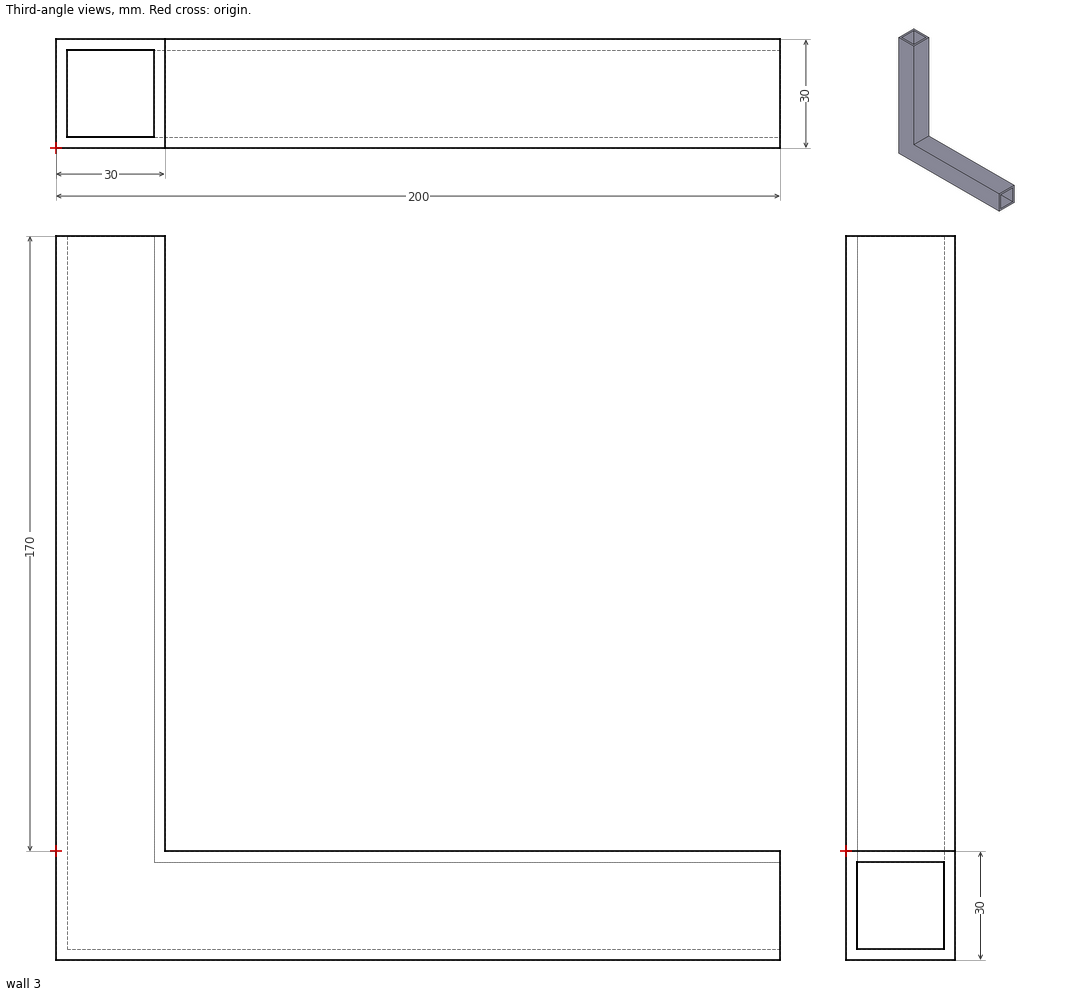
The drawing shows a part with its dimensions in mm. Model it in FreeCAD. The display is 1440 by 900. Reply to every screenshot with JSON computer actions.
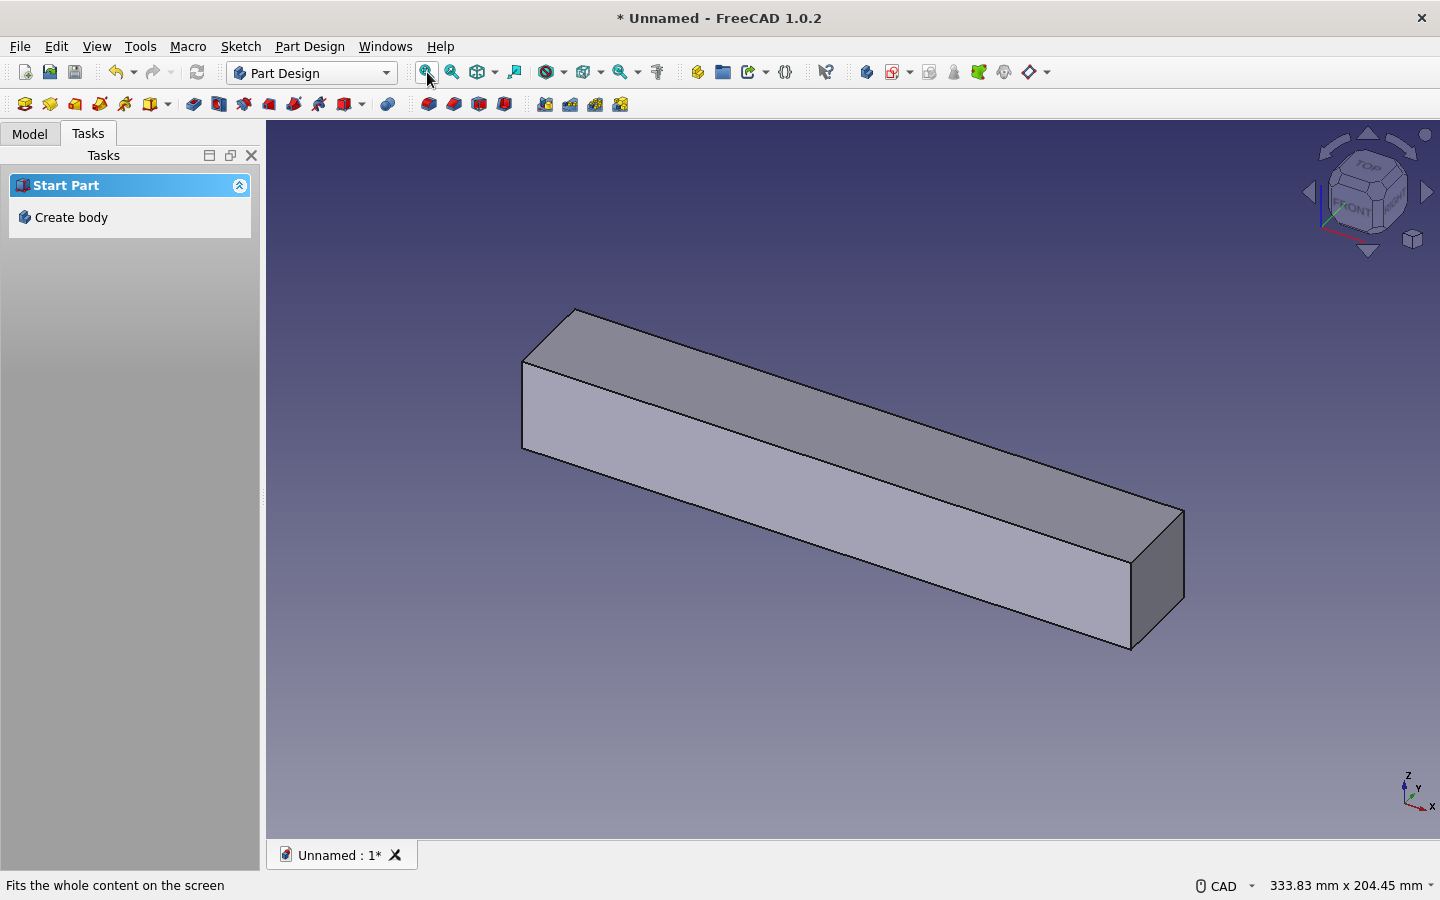
{"action": "left_click", "coordinate": [892, 72]}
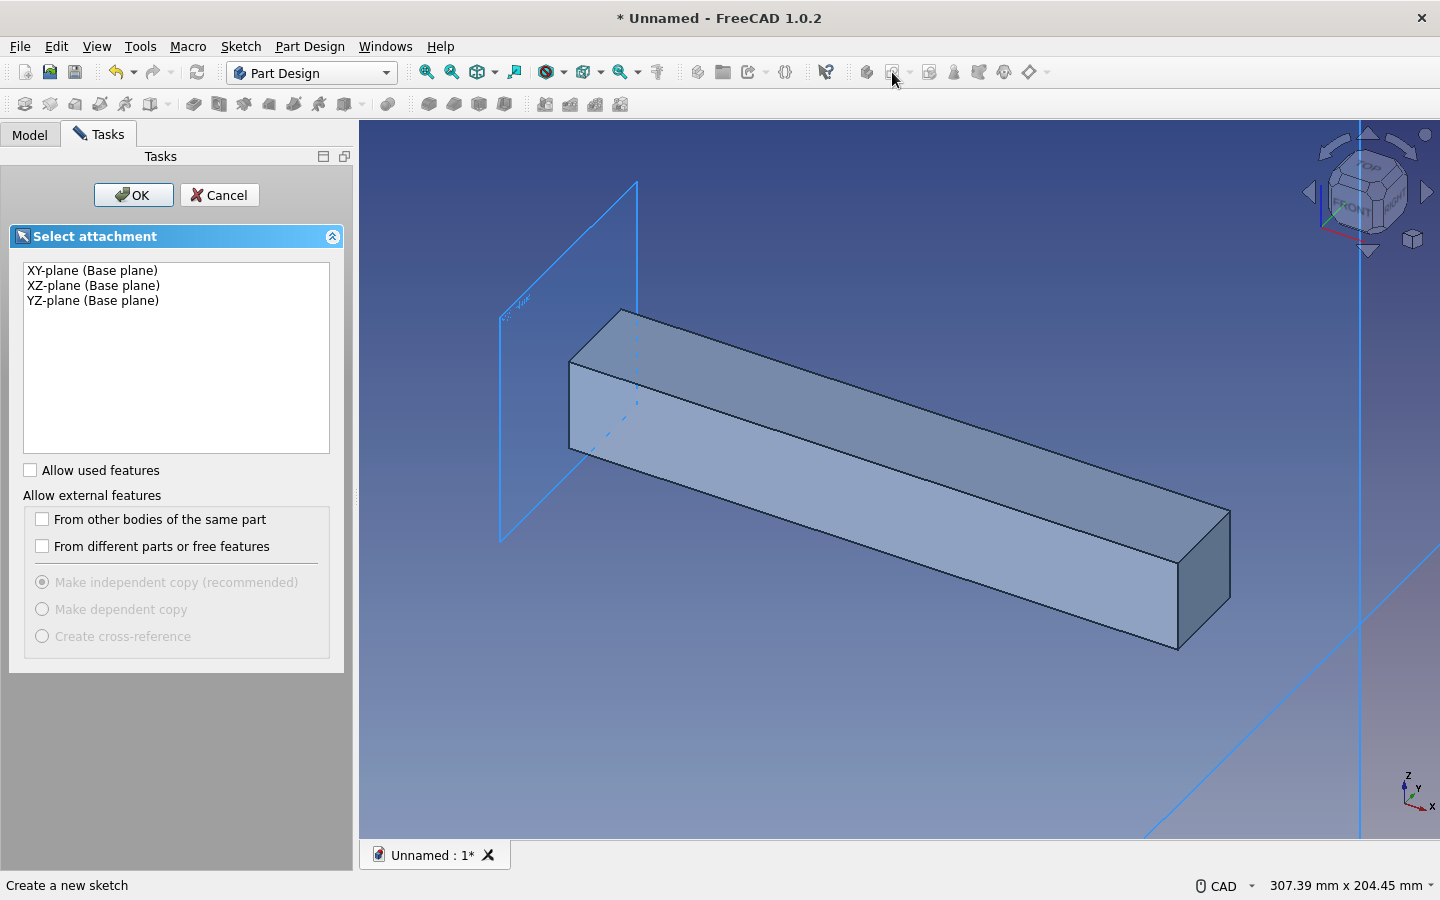
{"action": "left_click", "coordinate": [84, 270]}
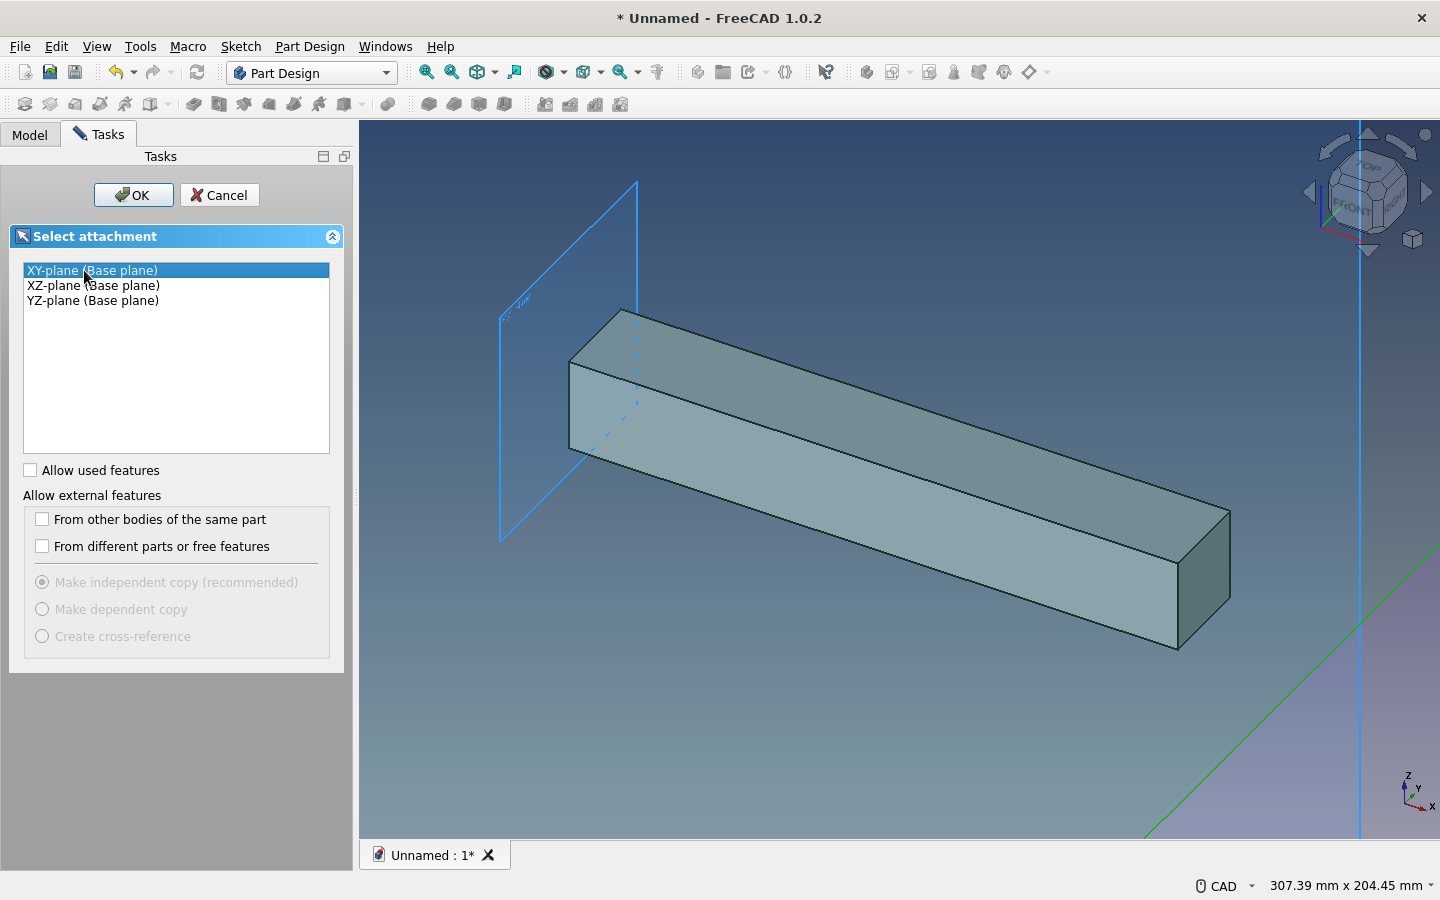
{"action": "left_click", "coordinate": [134, 195]}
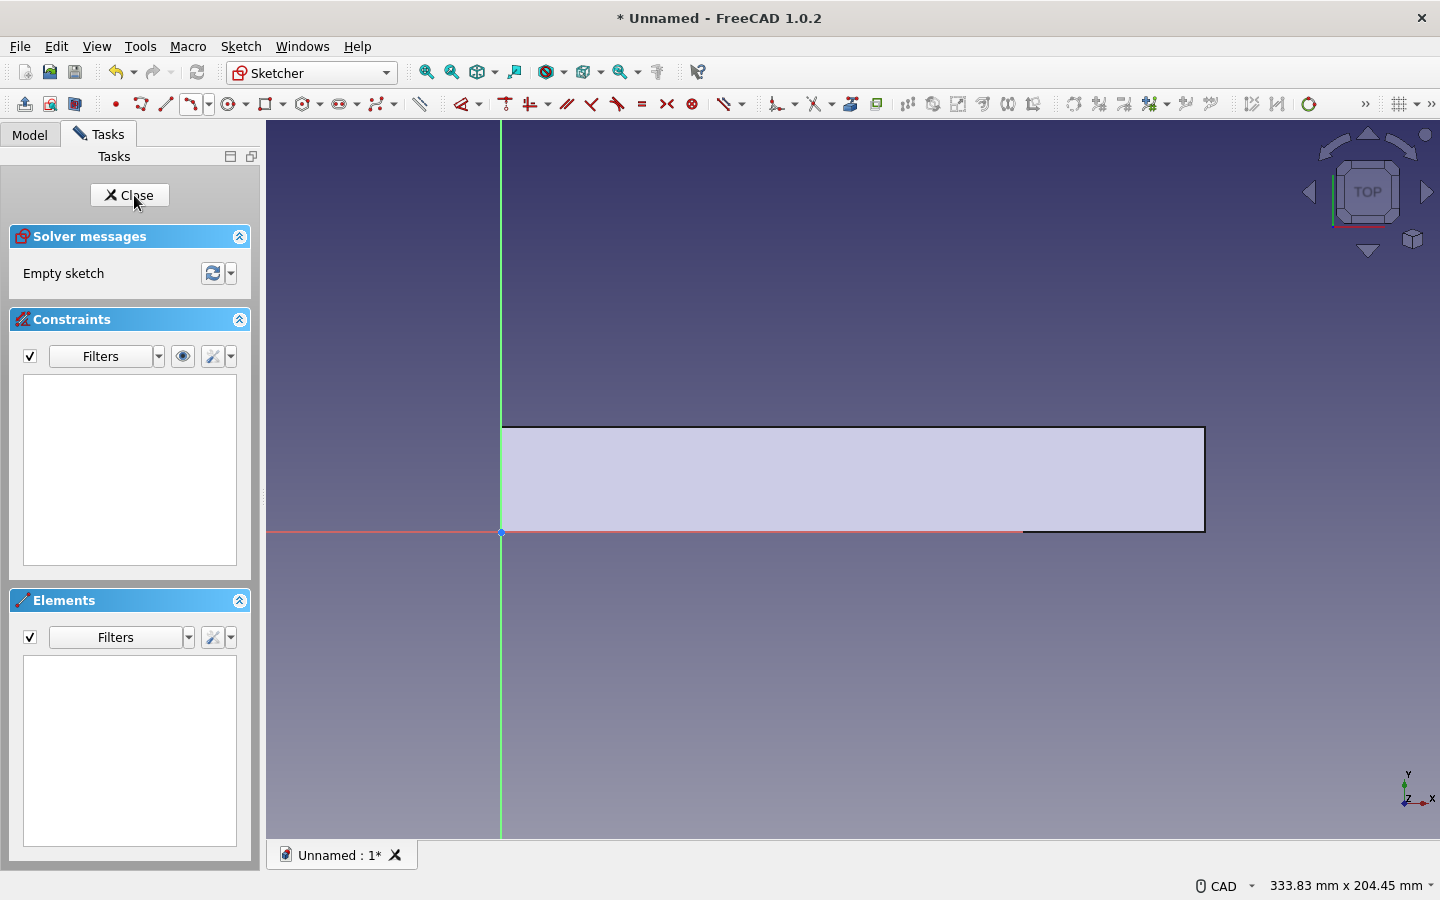
{"action": "scroll", "coordinate": [479, 480], "scroll_direction": "up", "scroll_amount": 7}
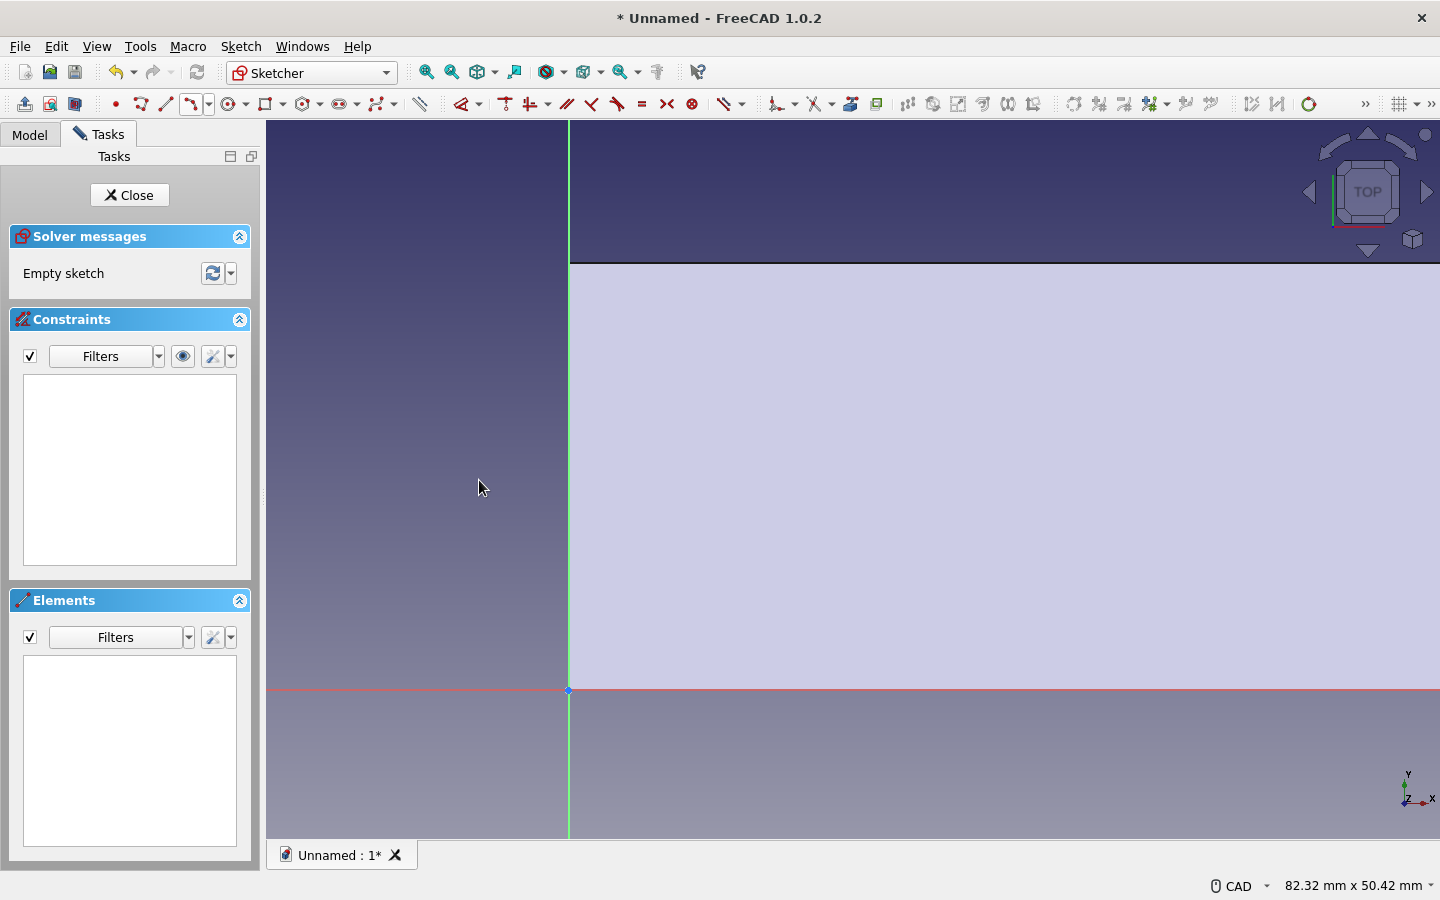
{"action": "left_click", "coordinate": [264, 104]}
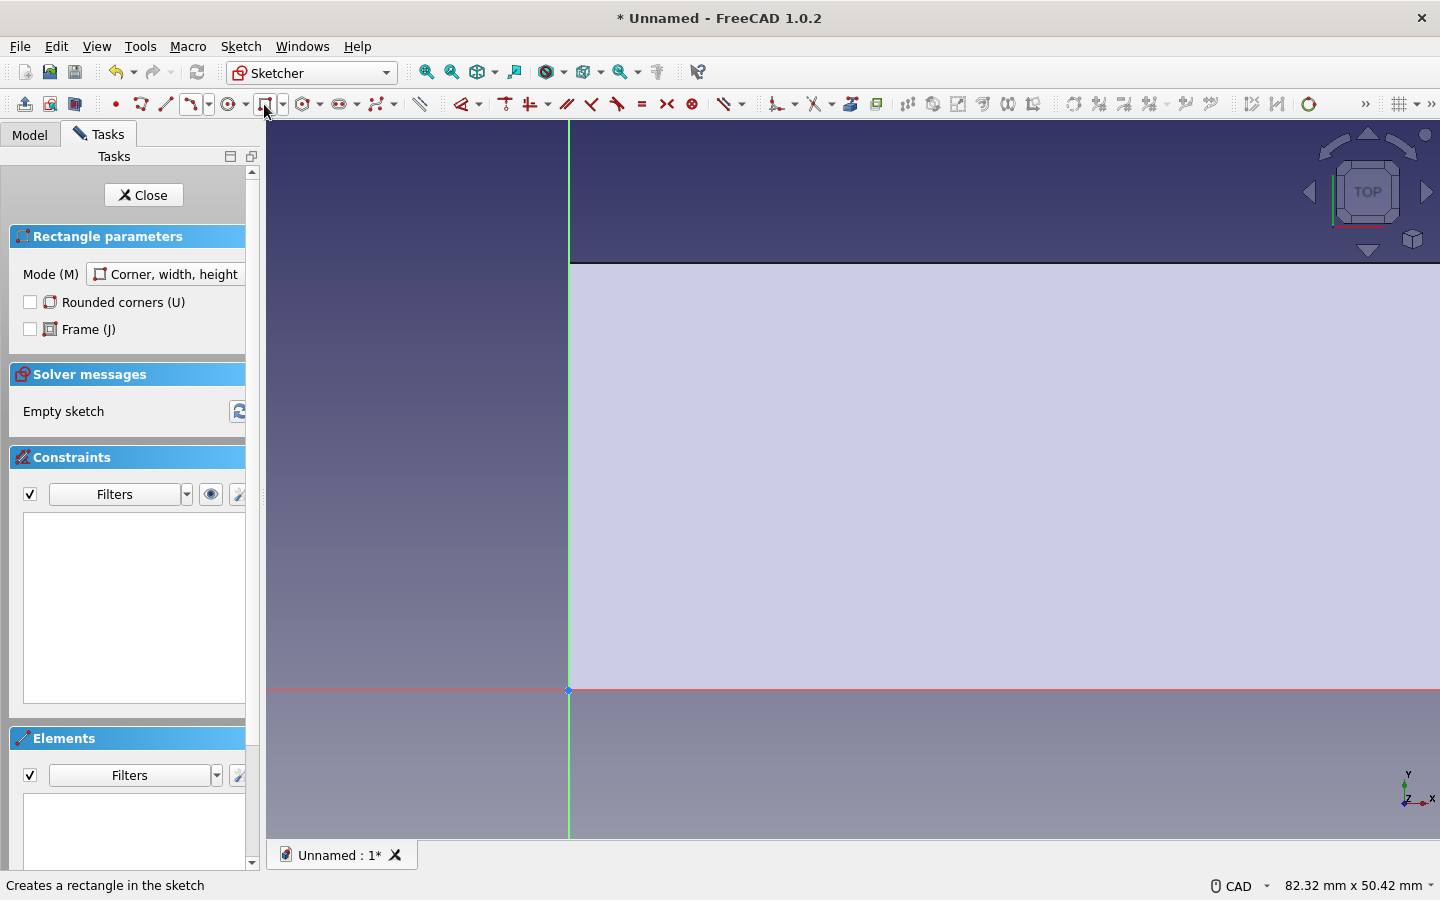
{"action": "left_click", "coordinate": [569, 690]}
{"action": "mouse_move", "coordinate": [997, 263]}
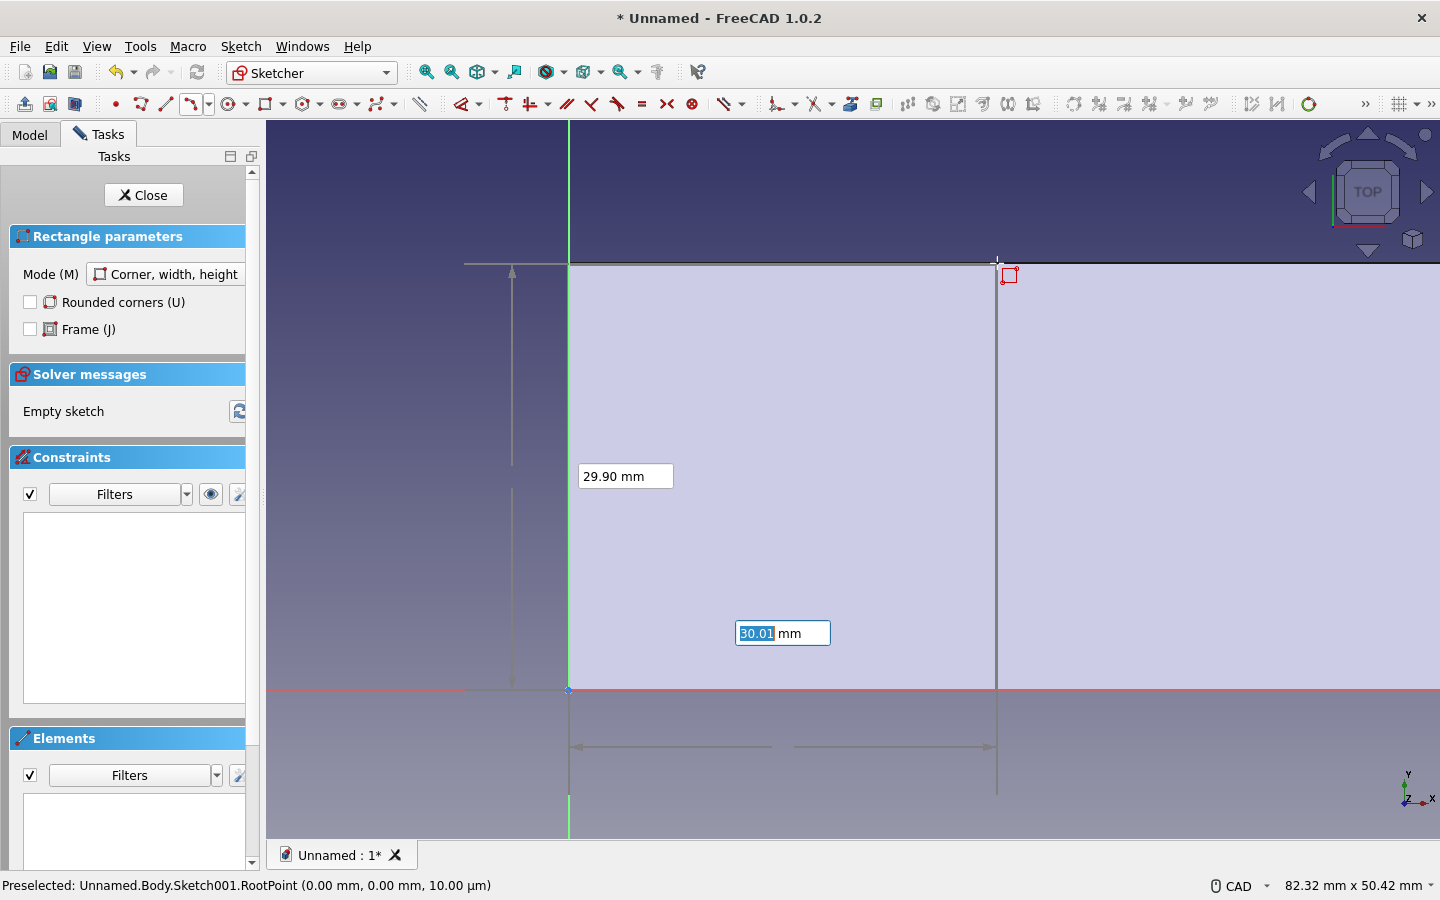
{"action": "type", "text": "30"}
{"action": "key", "text": "Tab"}
{"action": "type", "text": "30"}
{"action": "key", "text": "Return"}
{"action": "key", "text": "Escape"}